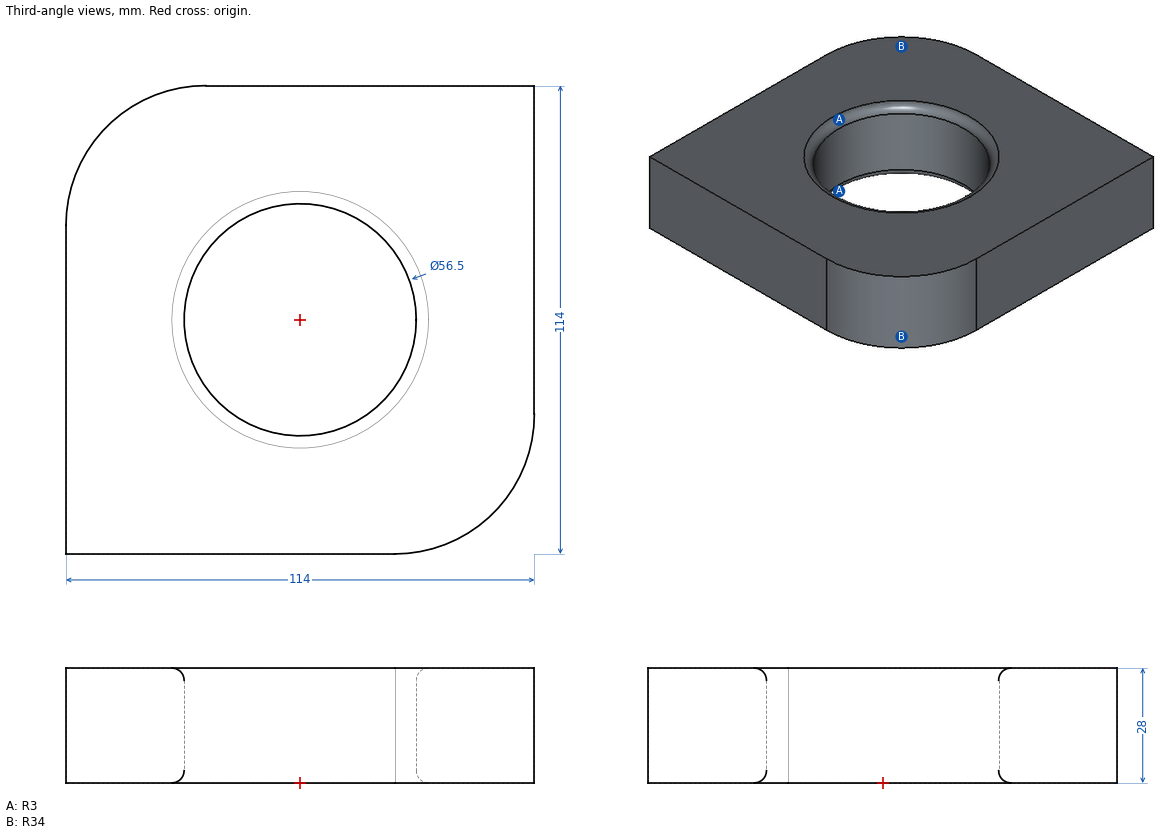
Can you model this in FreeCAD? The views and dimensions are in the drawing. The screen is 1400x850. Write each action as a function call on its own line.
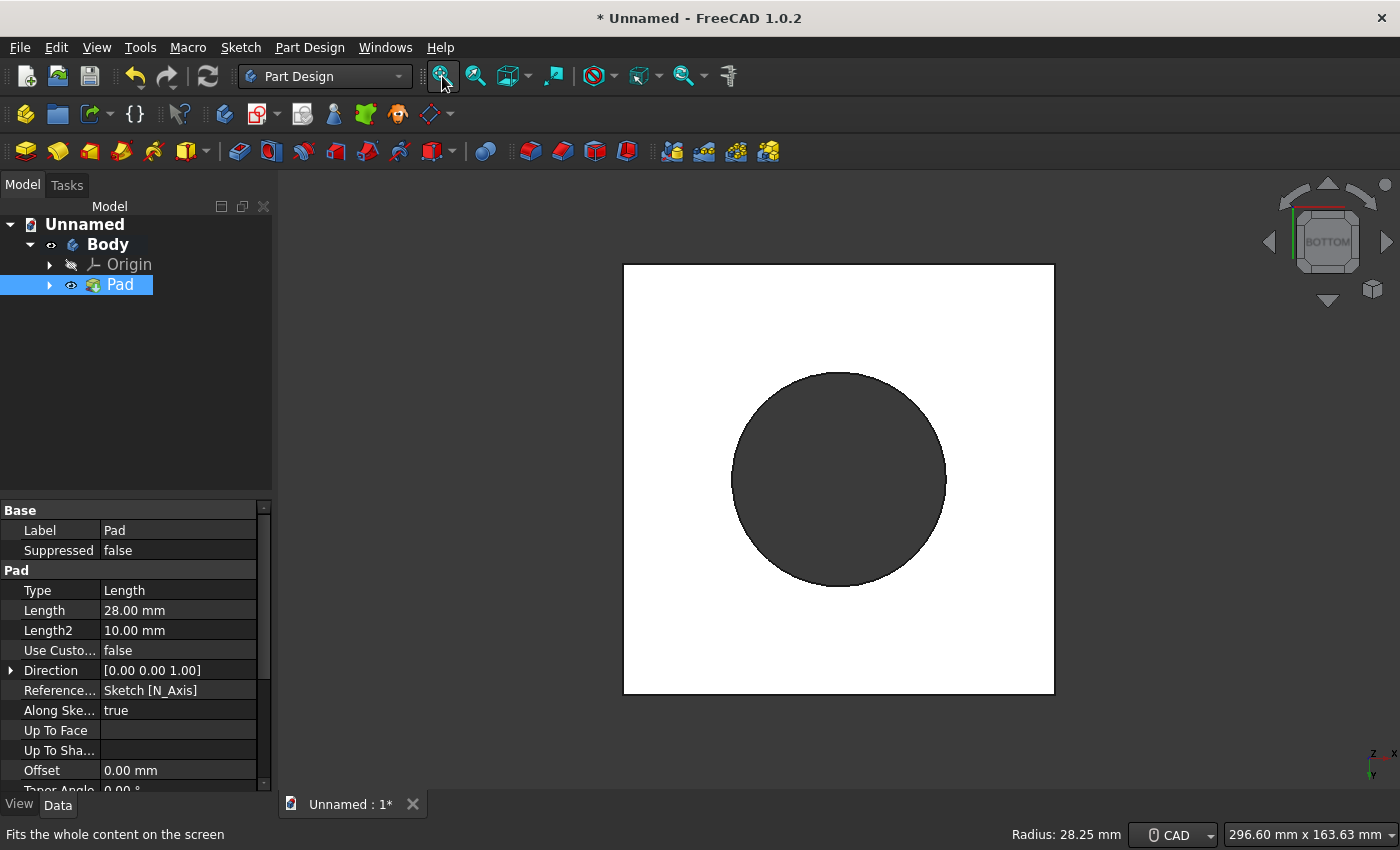
click(732, 478, ctrl)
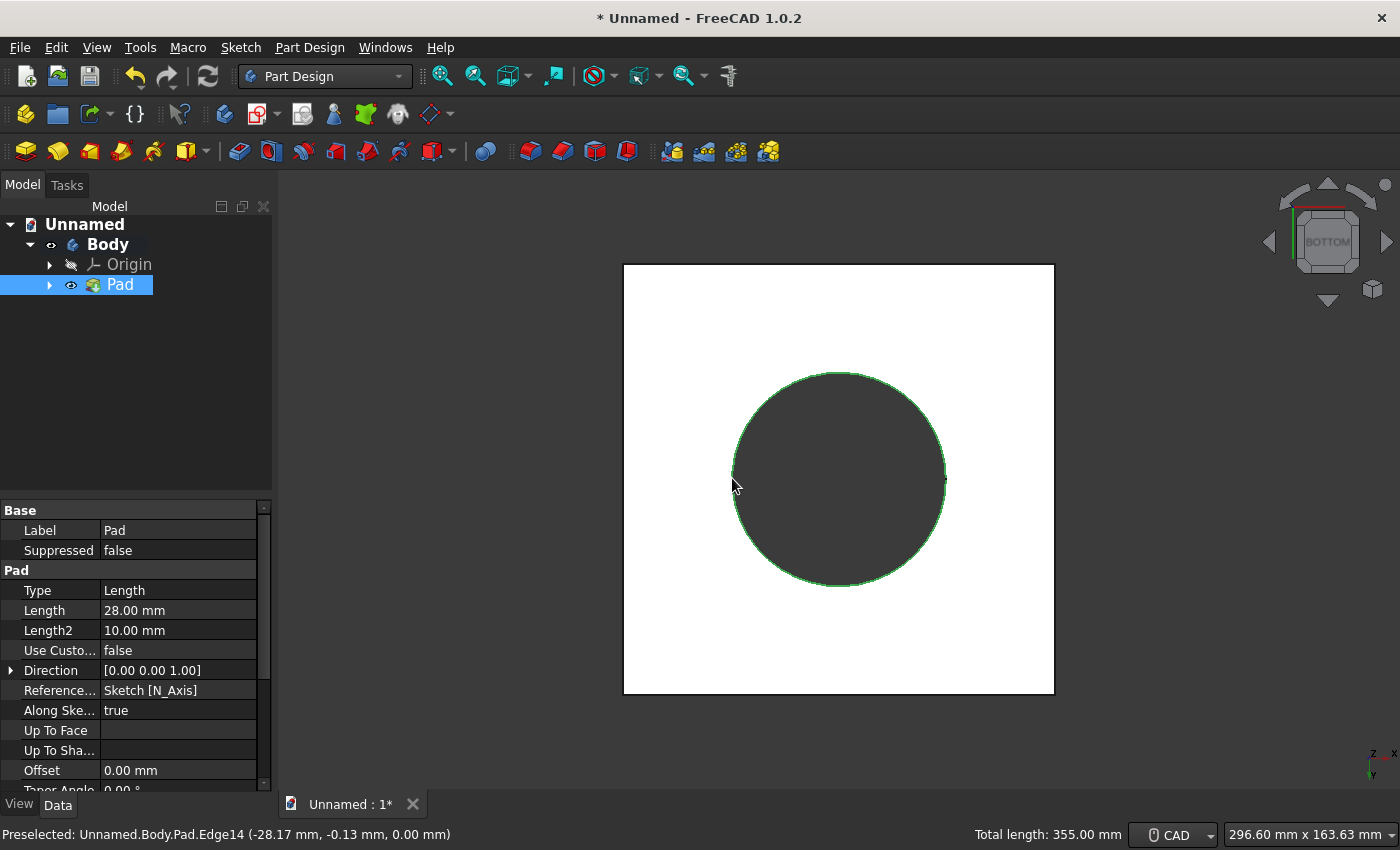
click(532, 152)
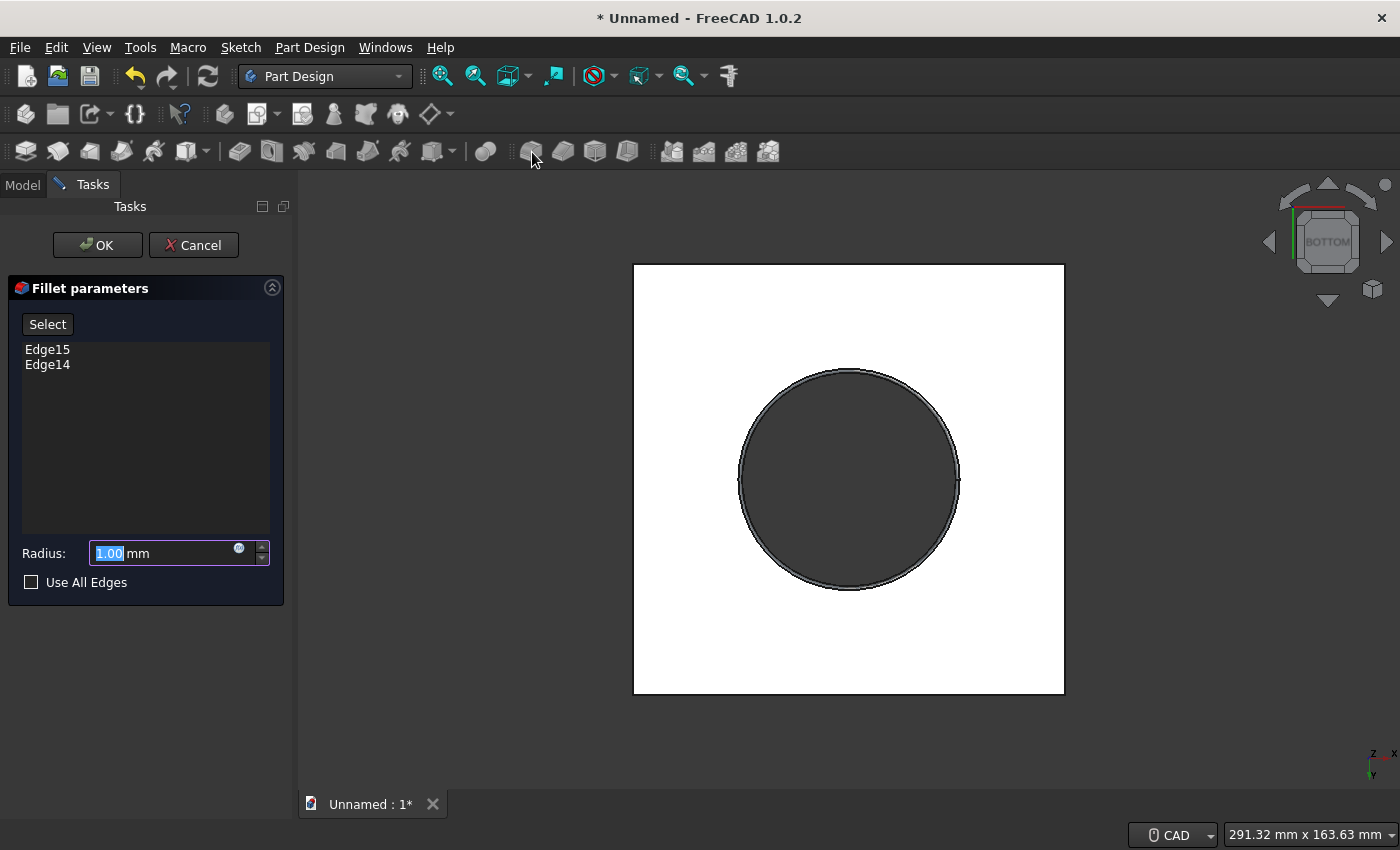
text(3)
key(Tab)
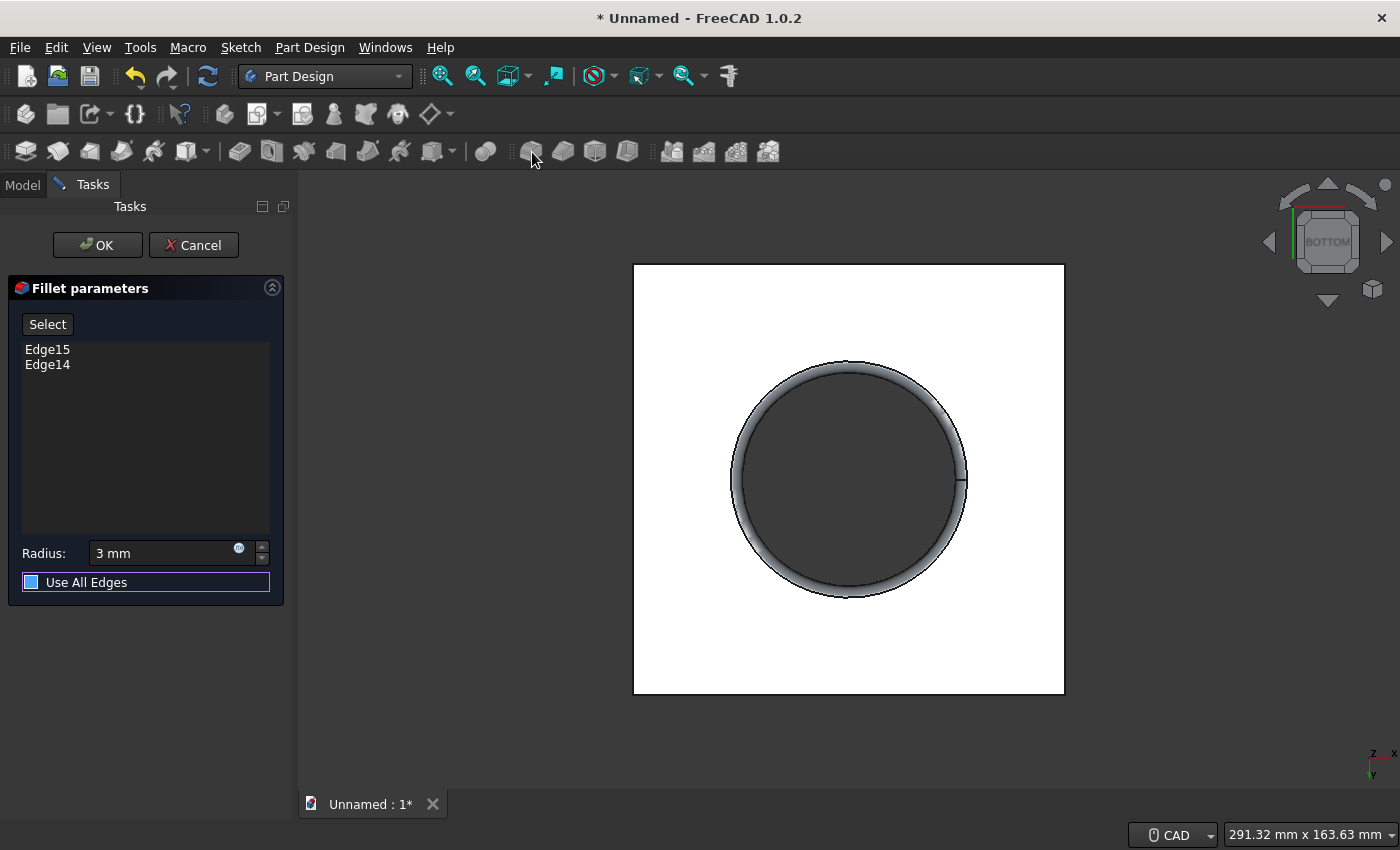
click(98, 245)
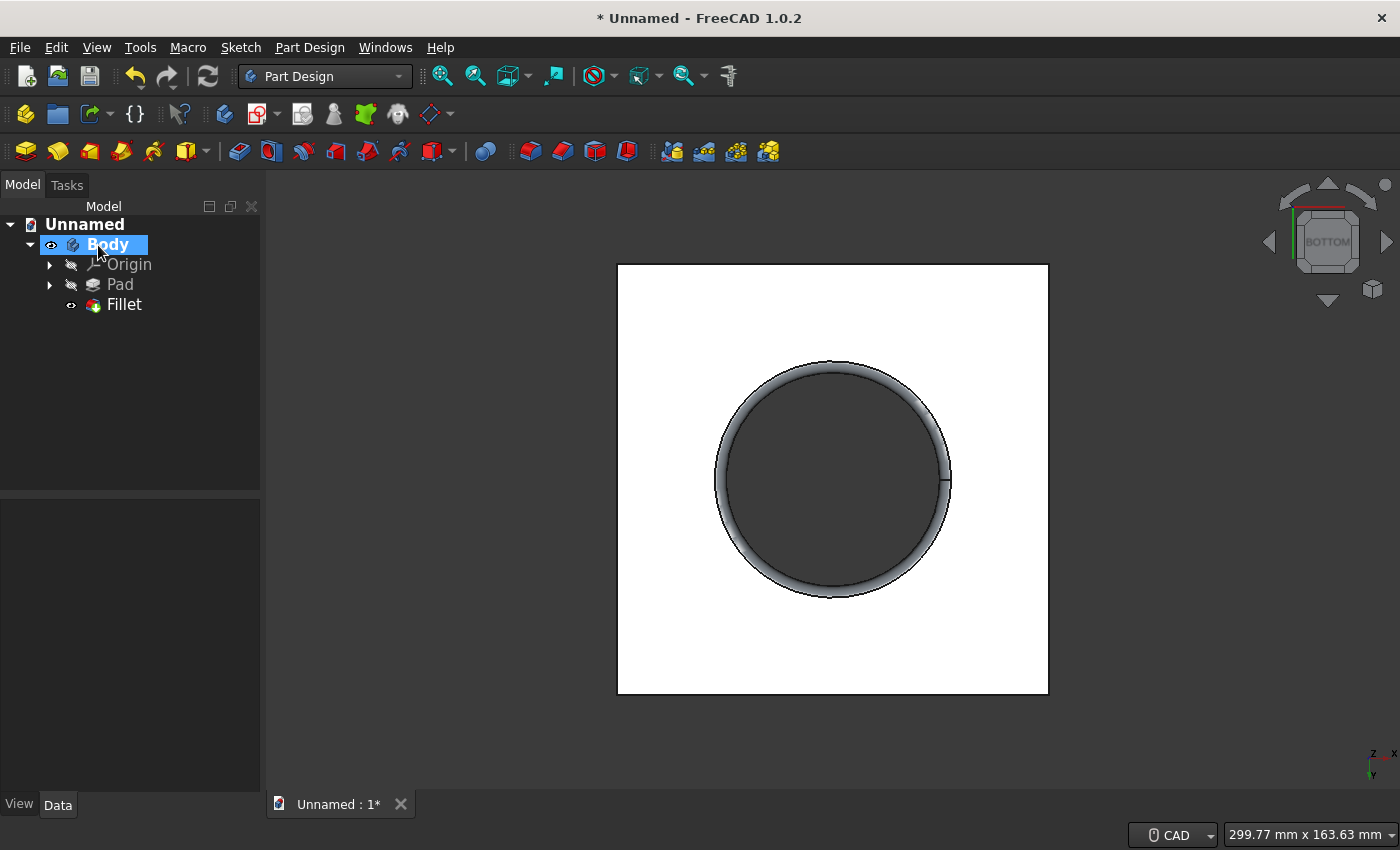
key(0)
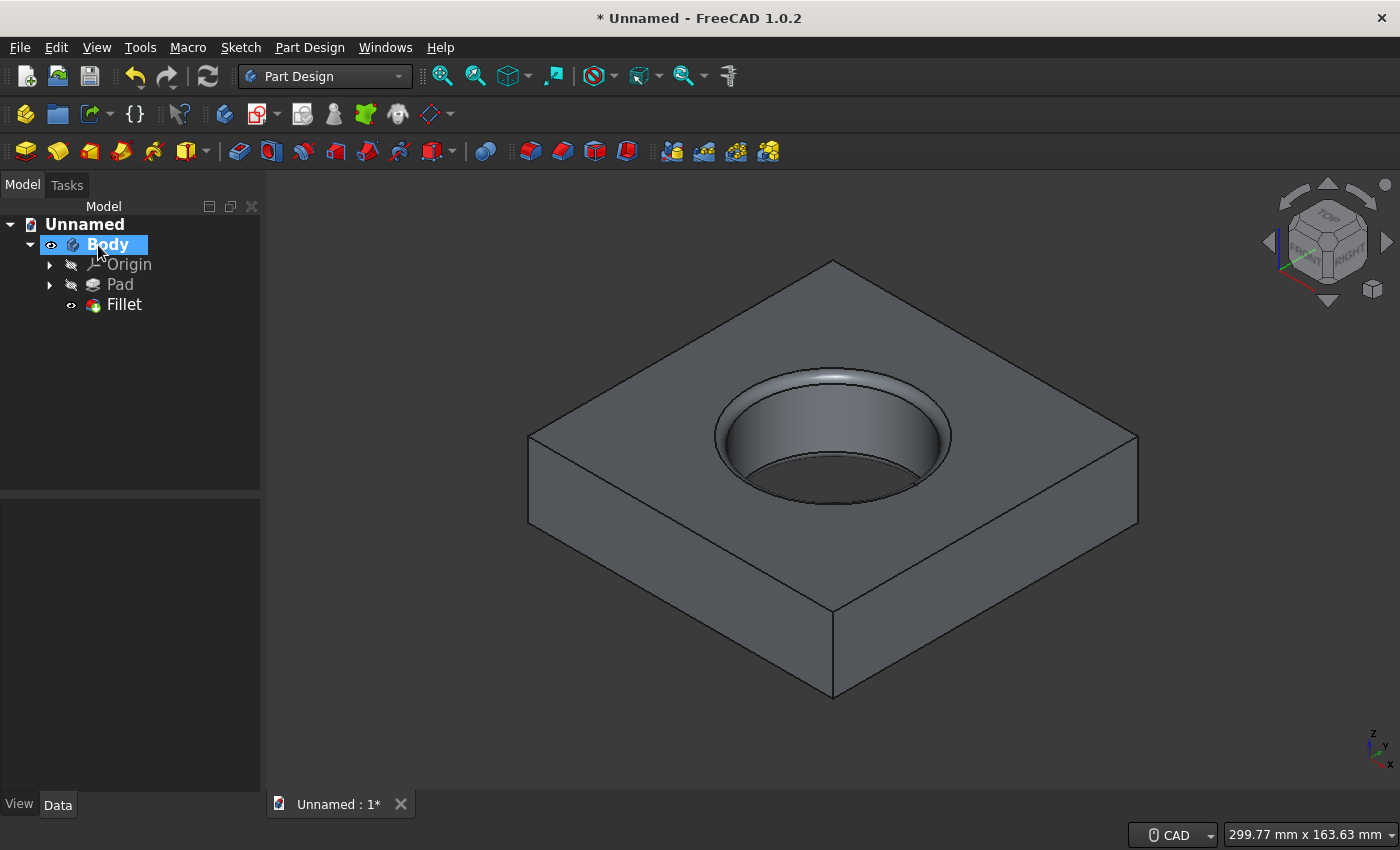
click(833, 655)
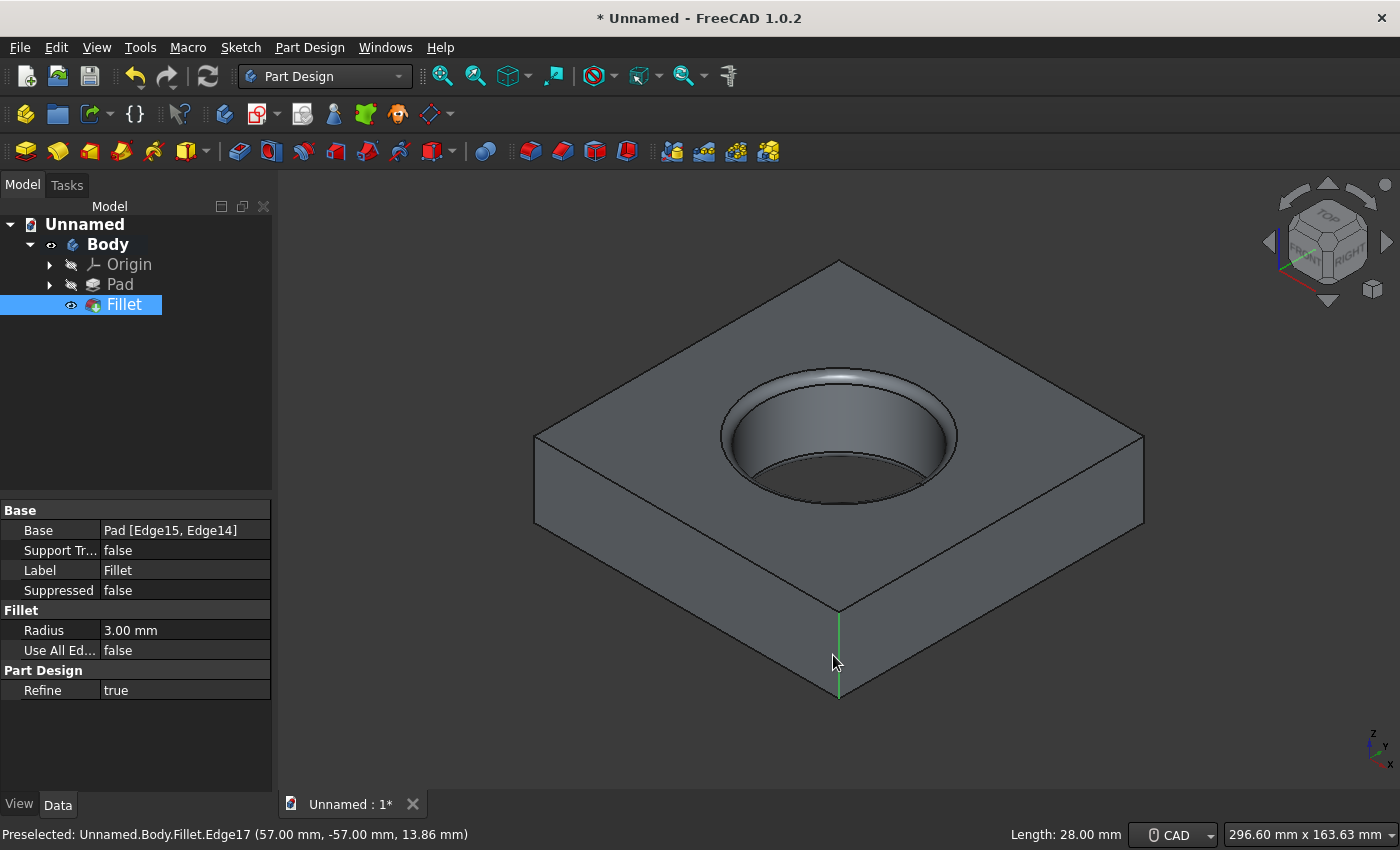
key(2)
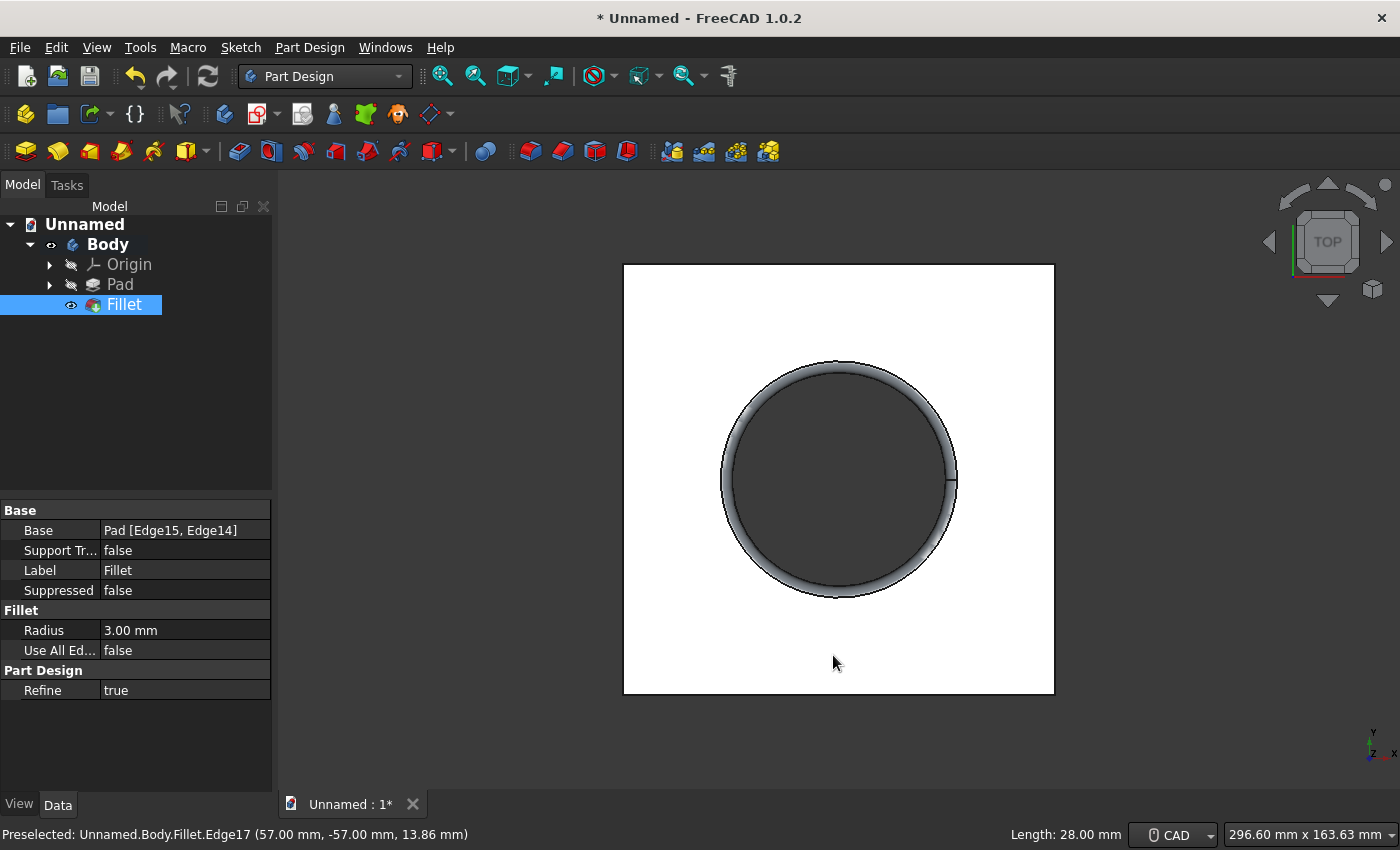
key(1)